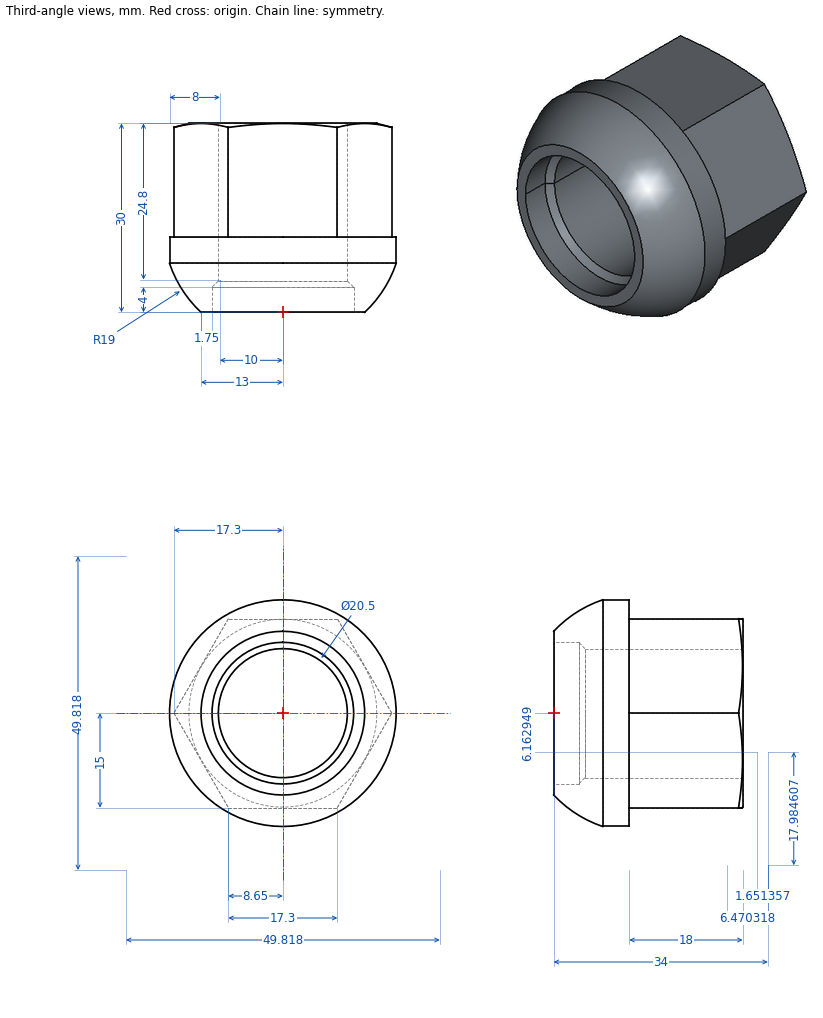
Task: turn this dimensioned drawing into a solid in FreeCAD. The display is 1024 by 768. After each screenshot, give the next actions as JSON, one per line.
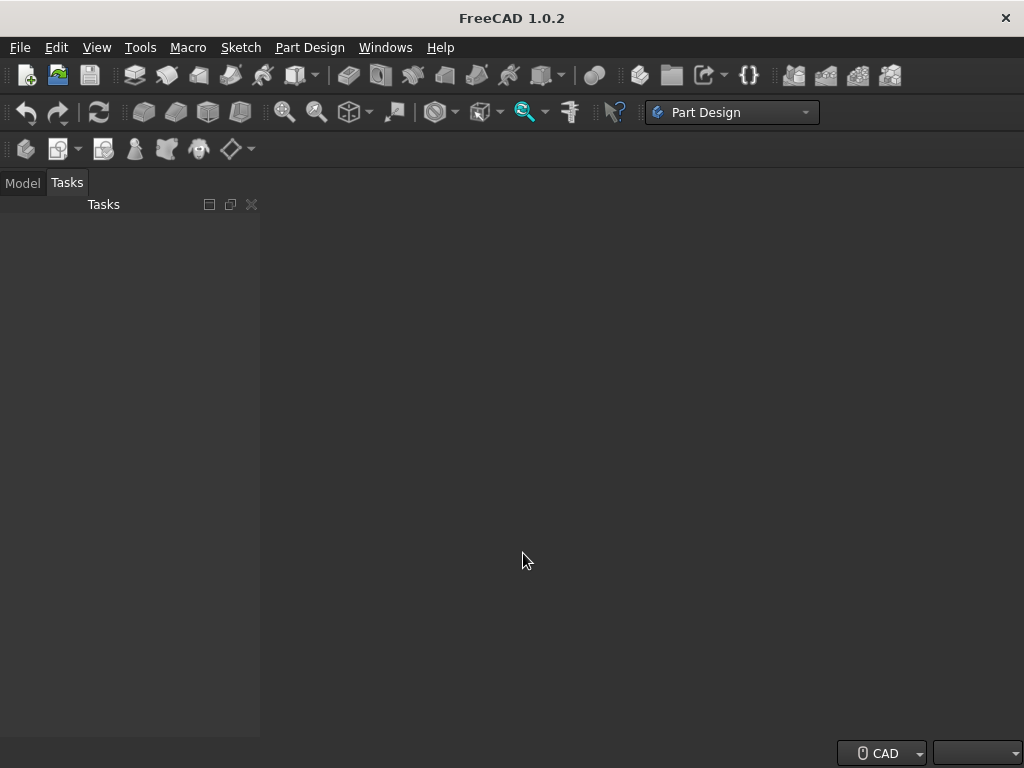
{"action": "left_click", "coordinate": [26, 76]}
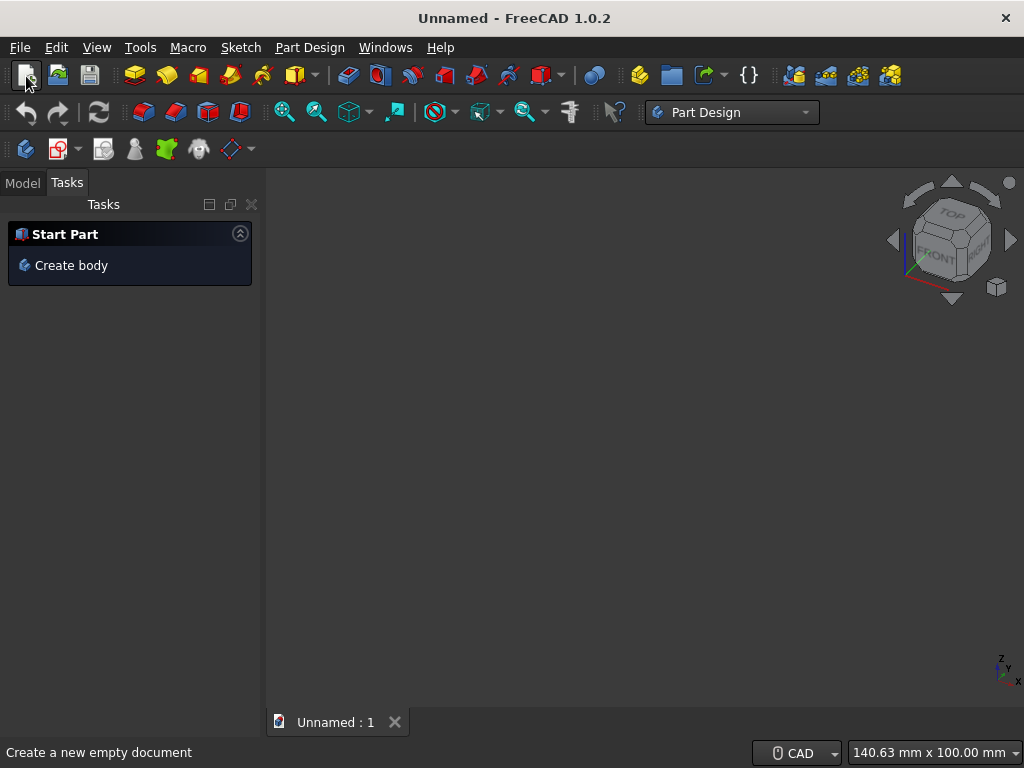
{"action": "left_click", "coordinate": [58, 150]}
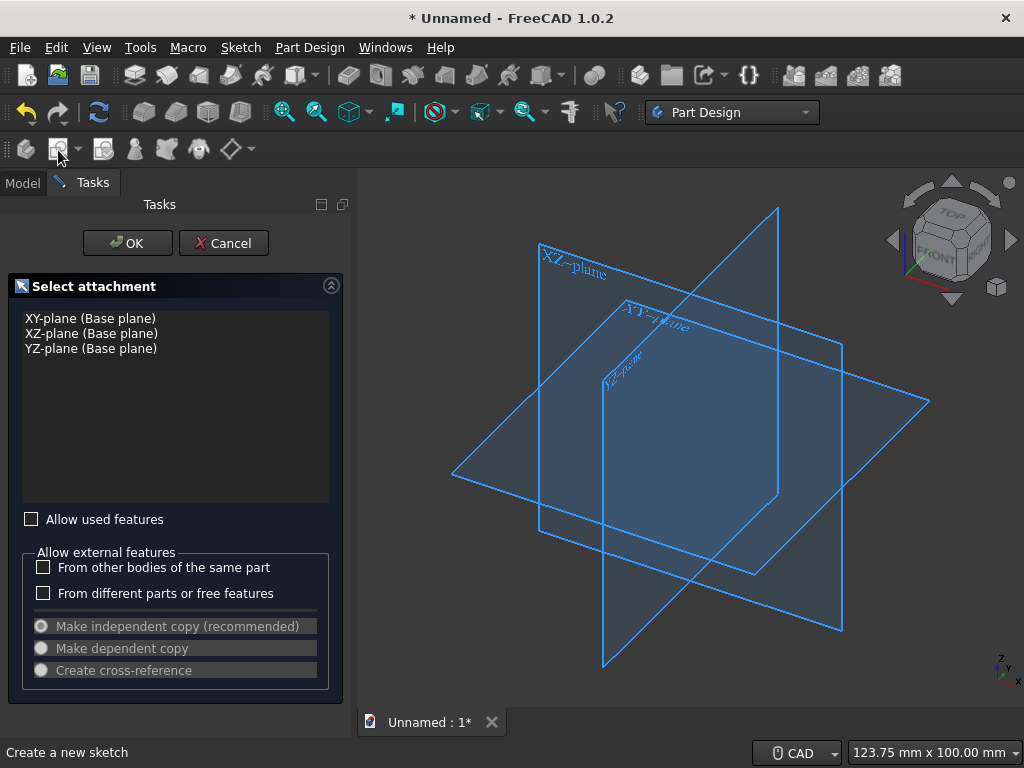
{"action": "left_click", "coordinate": [82, 318]}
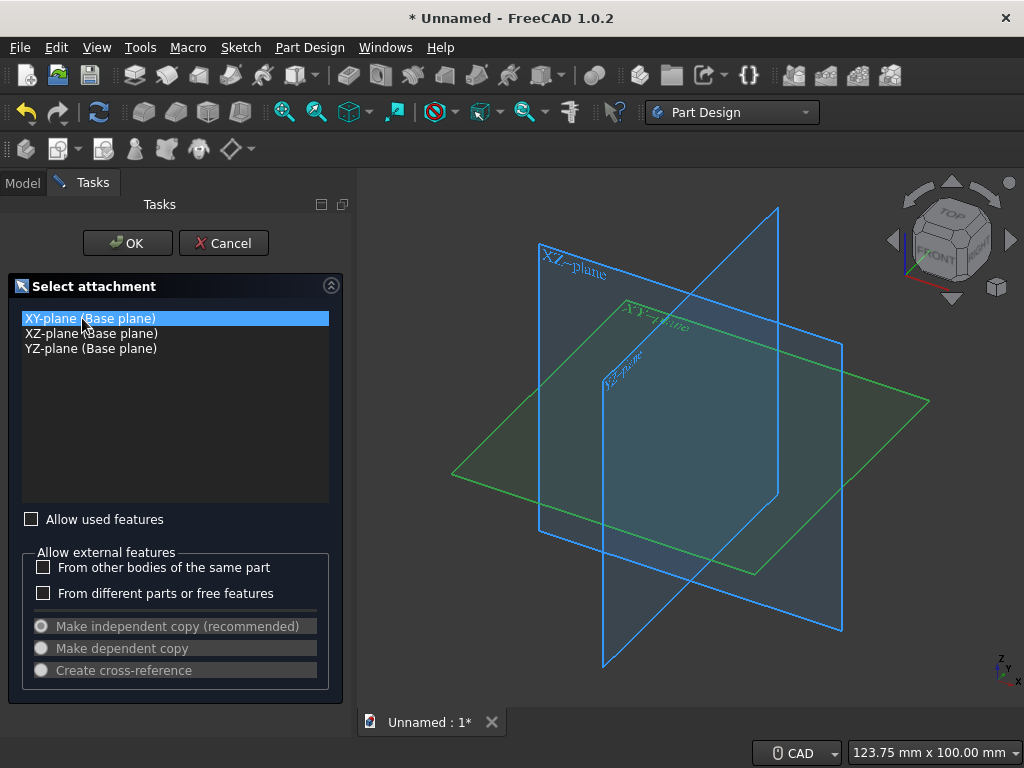
{"action": "left_click", "coordinate": [128, 243]}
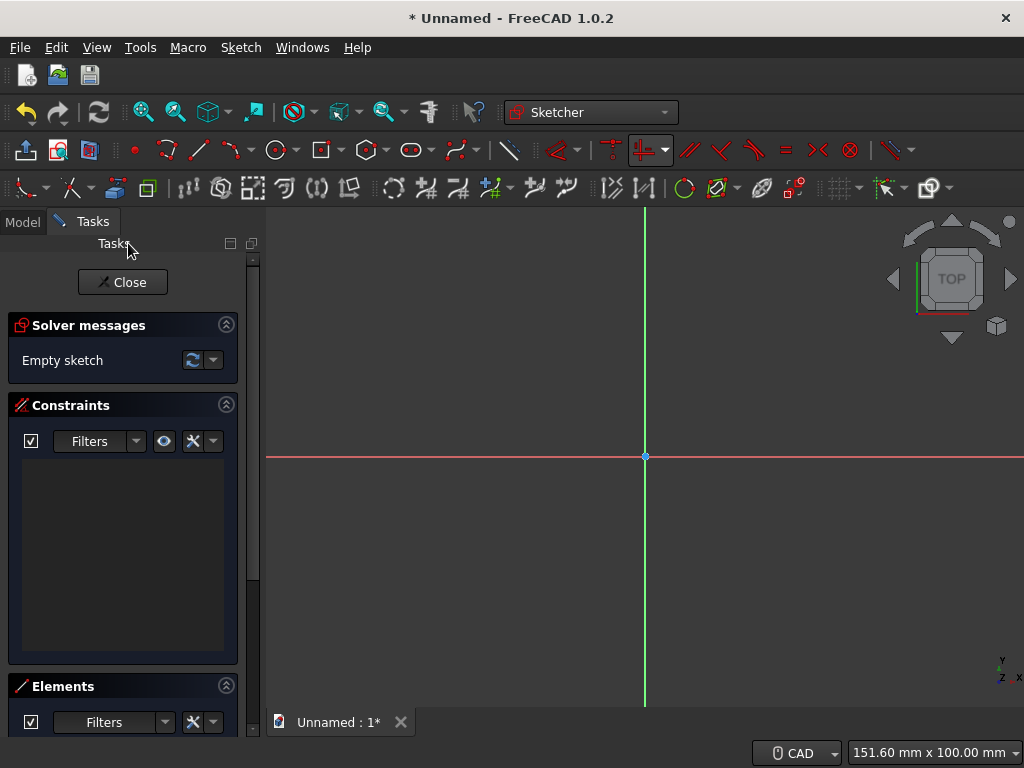
{"action": "scroll", "coordinate": [619, 321], "scroll_direction": "up", "scroll_amount": 4}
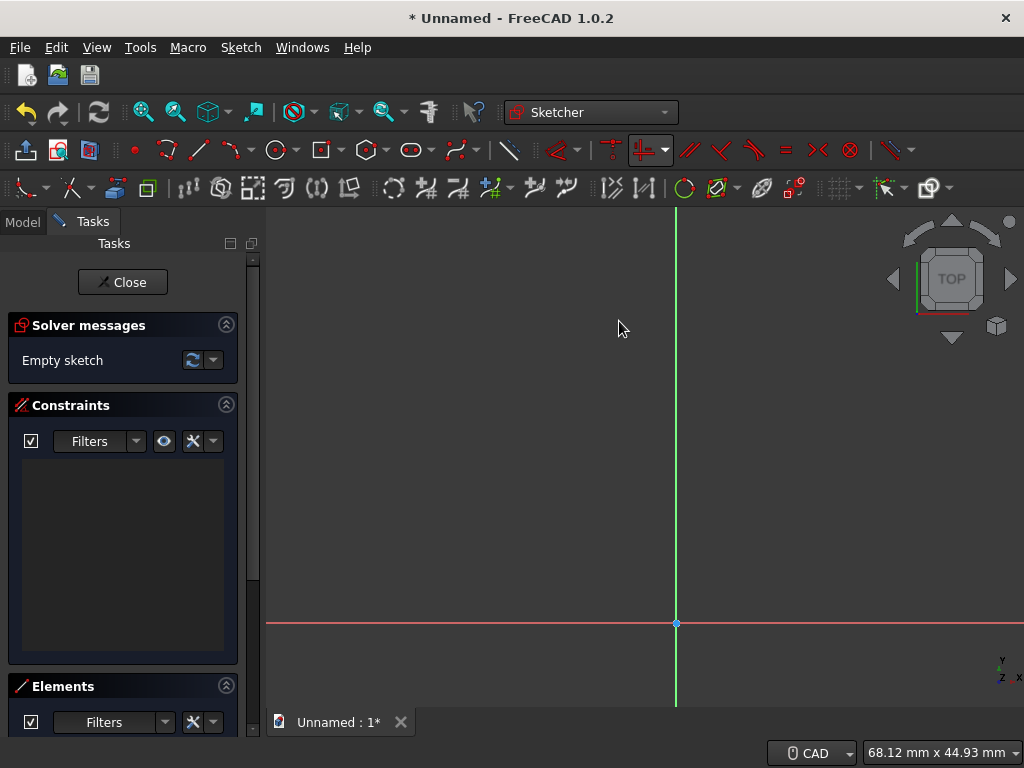
{"action": "left_click", "coordinate": [168, 150]}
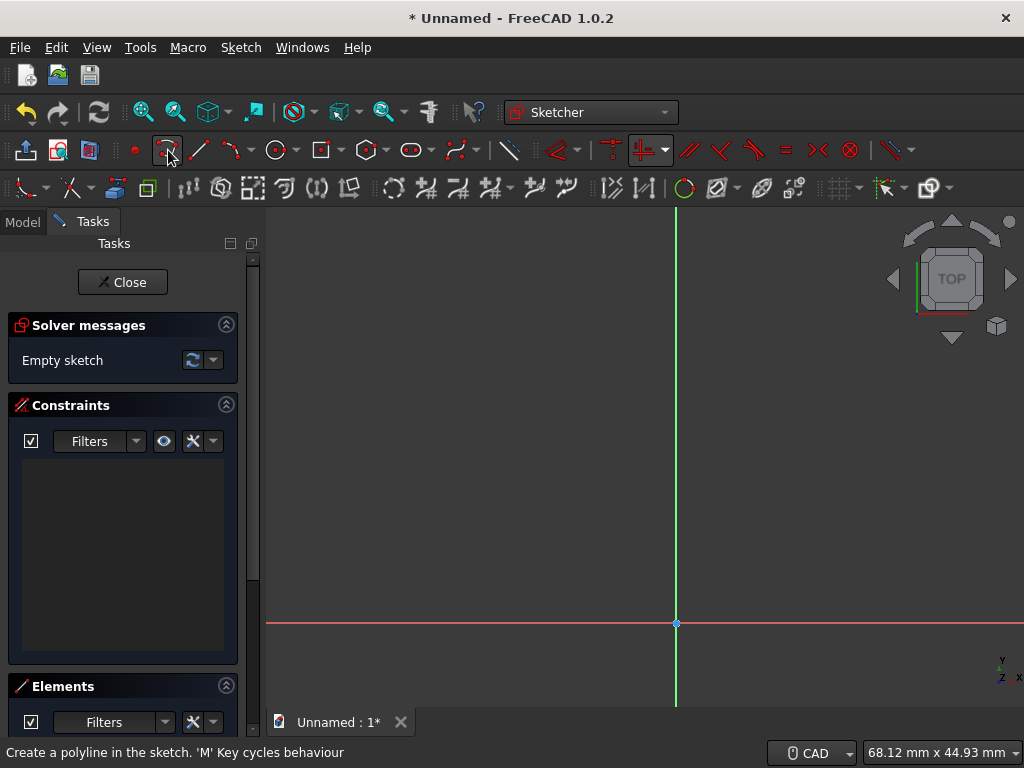
{"action": "left_click", "coordinate": [532, 623]}
{"action": "left_click", "coordinate": [551, 614]}
{"action": "left_click", "coordinate": [551, 579]}
{"action": "left_click", "coordinate": [565, 566]}
{"action": "left_click", "coordinate": [565, 290]}
{"action": "left_click", "coordinate": [476, 290]}
{"action": "left_click", "coordinate": [476, 537]}
{"action": "right_click", "coordinate": [476, 537]}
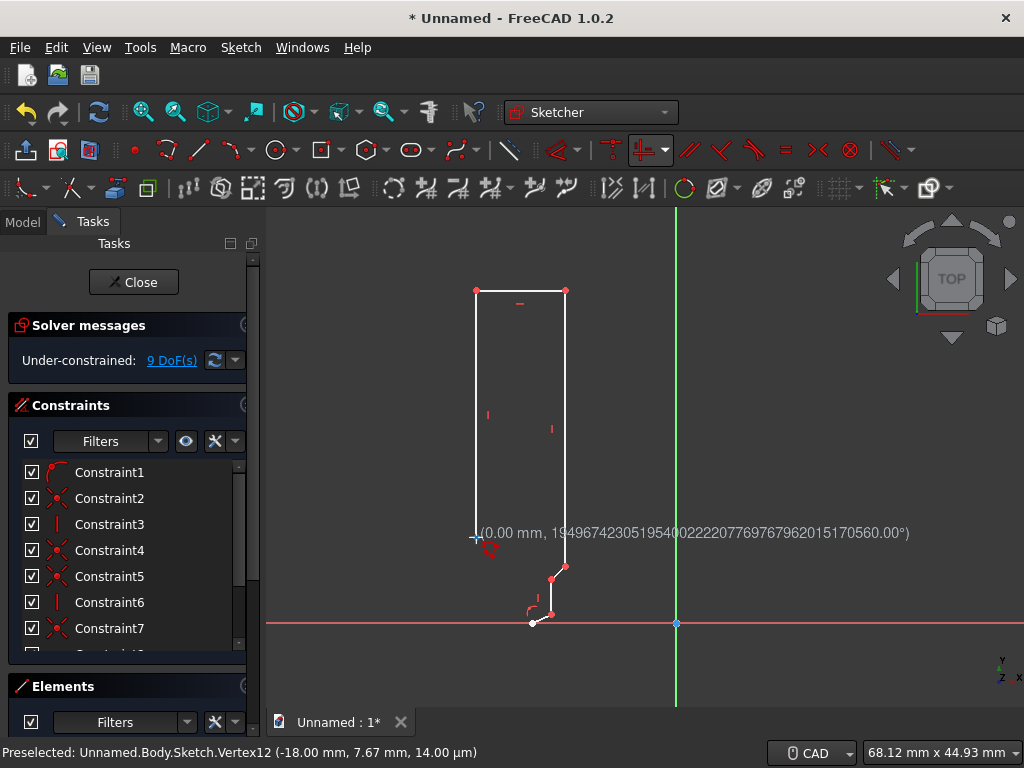
{"action": "key", "text": "g 3 a"}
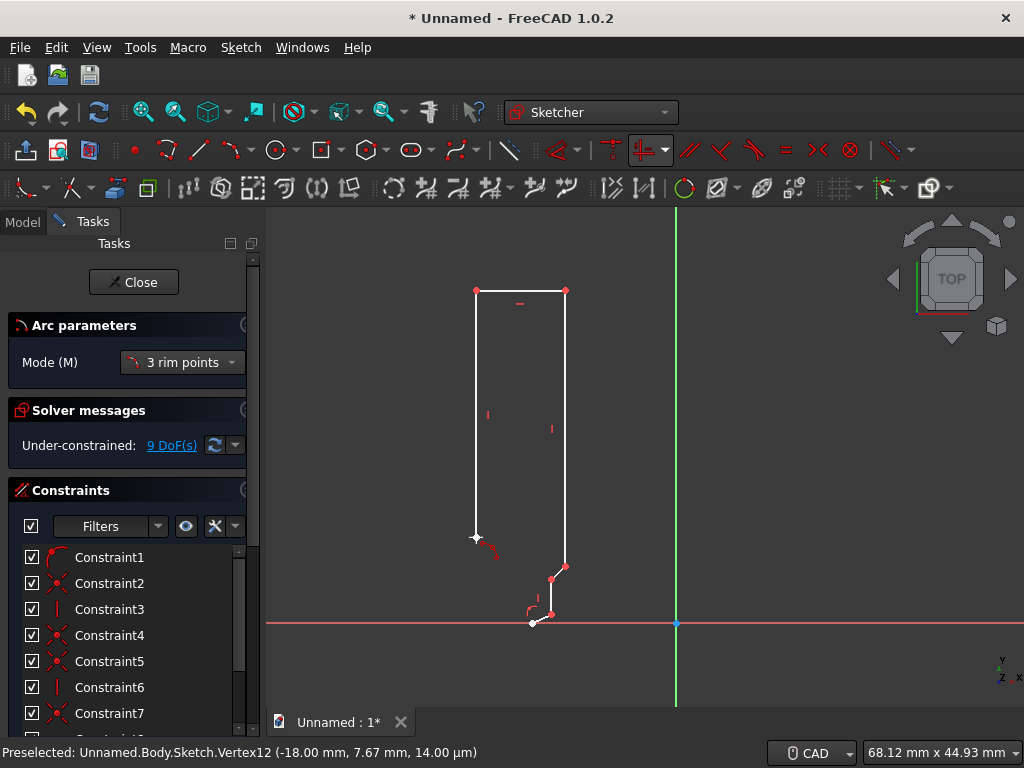
{"action": "left_click", "coordinate": [476, 538]}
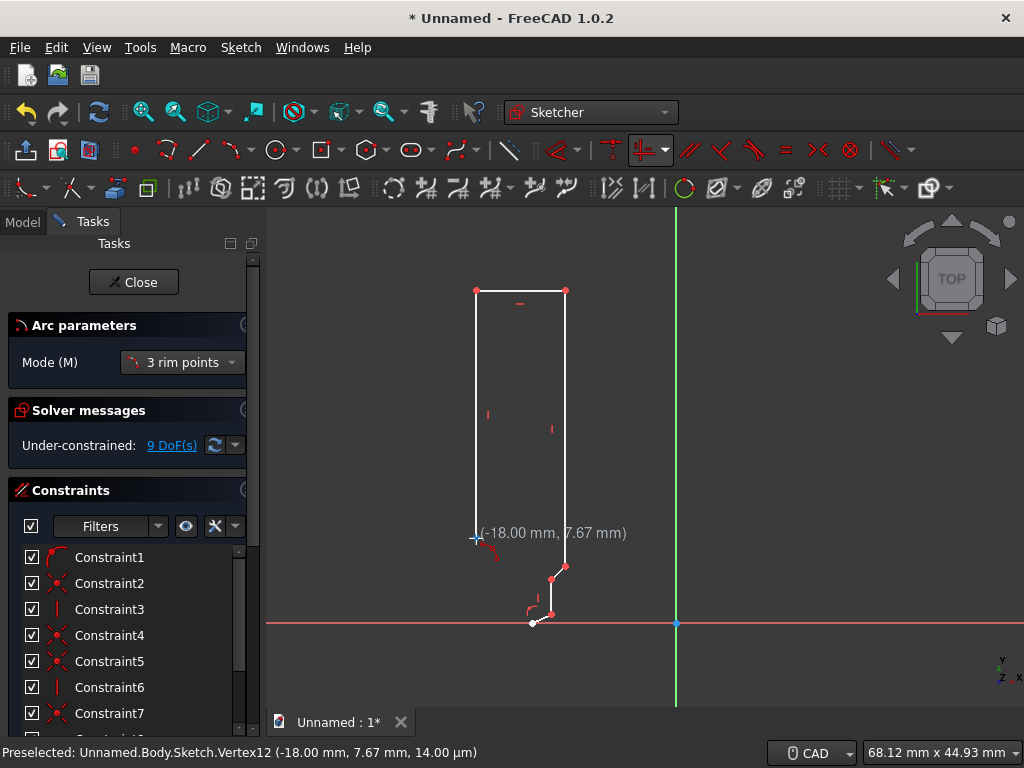
{"action": "scroll", "coordinate": [532, 623], "scroll_direction": "up", "scroll_amount": 3}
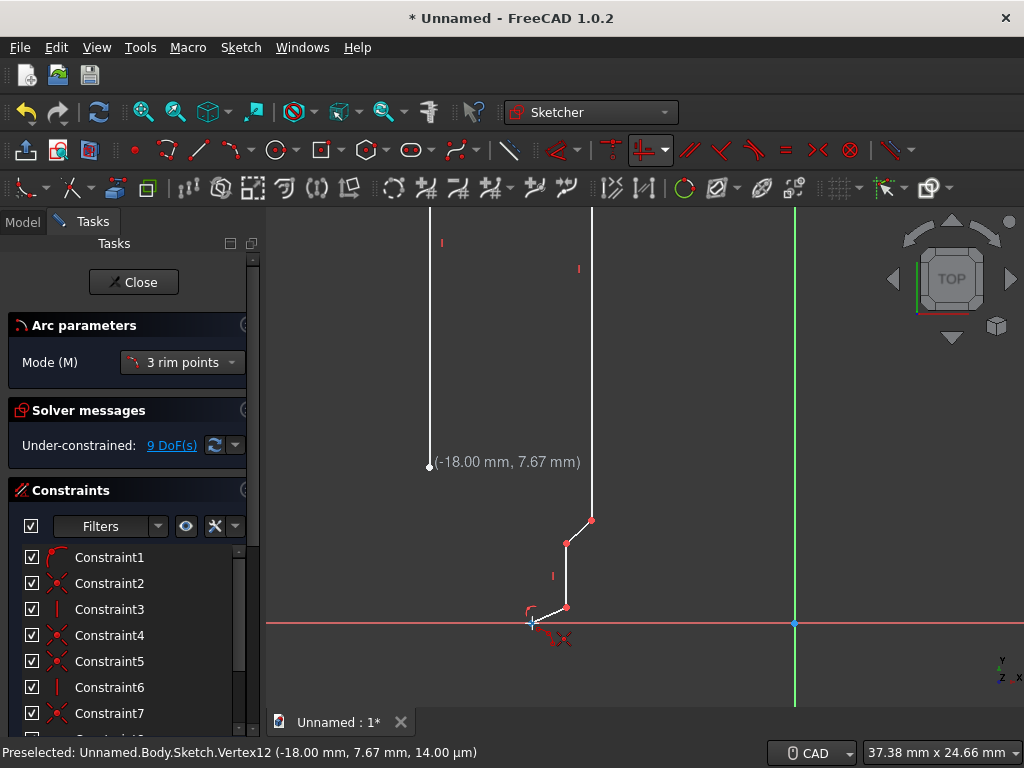
{"action": "left_click", "coordinate": [532, 623]}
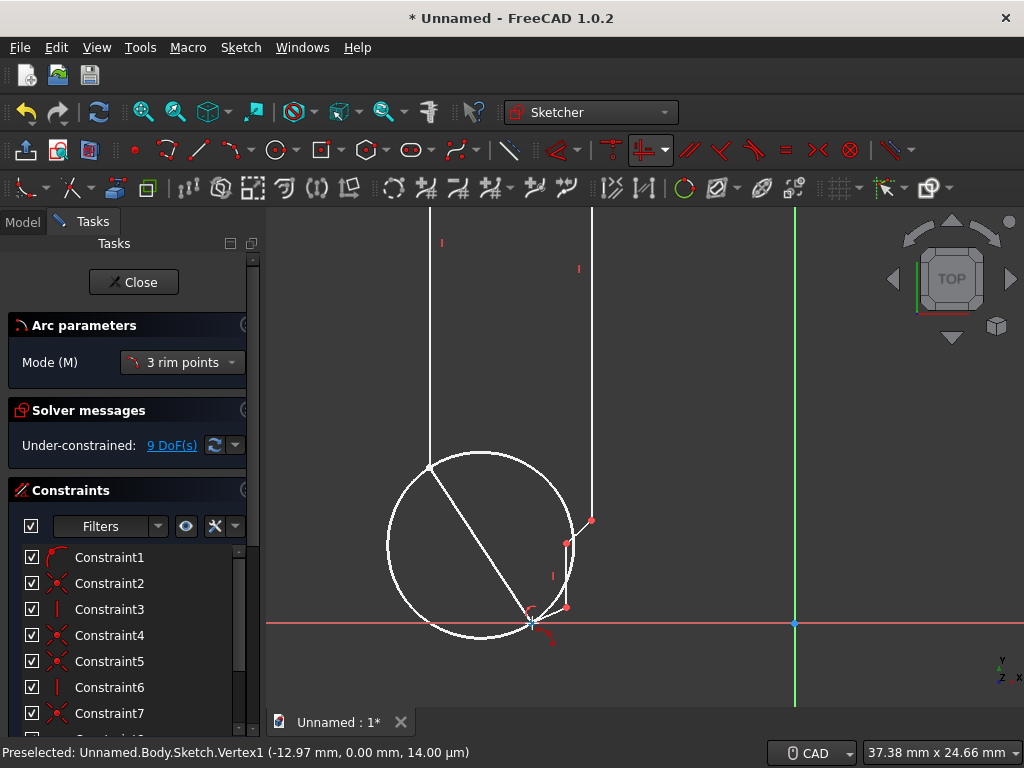
{"action": "scroll", "coordinate": [471, 550], "scroll_direction": "up", "scroll_amount": 2}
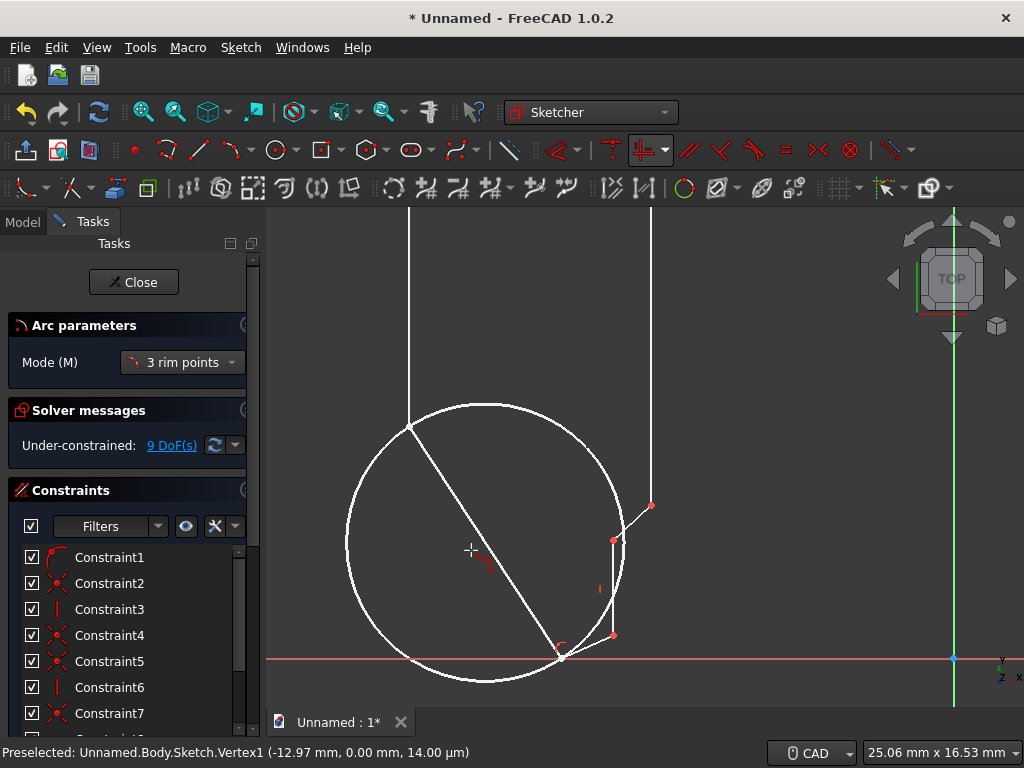
{"action": "left_click", "coordinate": [470, 550]}
{"action": "key", "text": "Escape"}